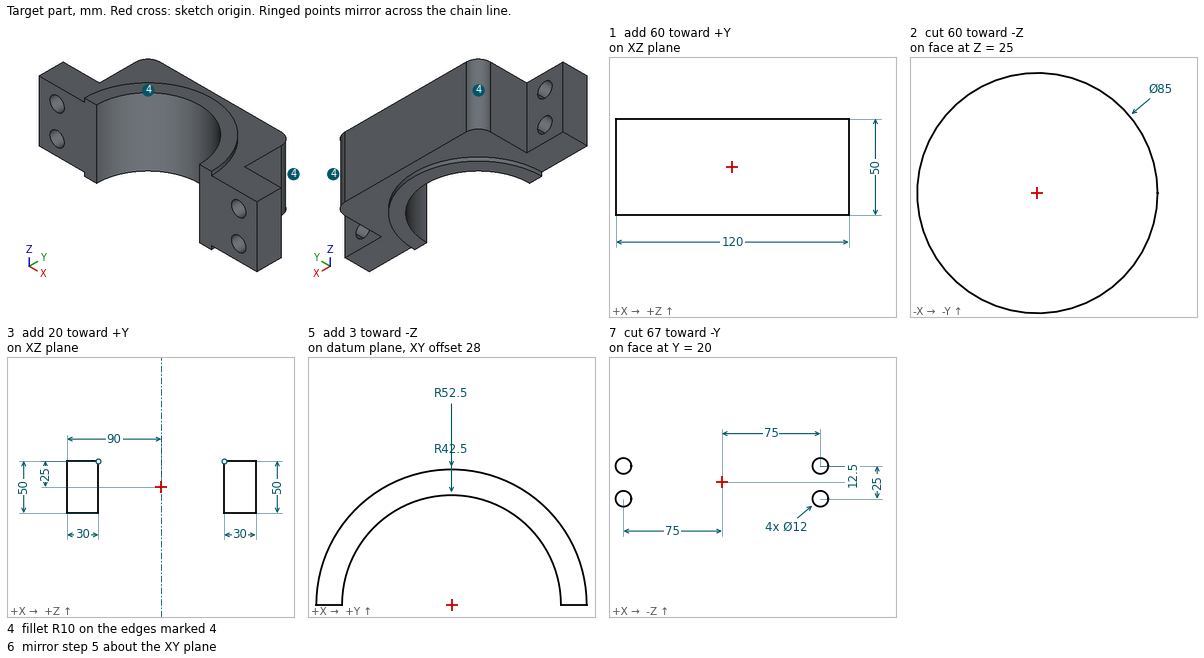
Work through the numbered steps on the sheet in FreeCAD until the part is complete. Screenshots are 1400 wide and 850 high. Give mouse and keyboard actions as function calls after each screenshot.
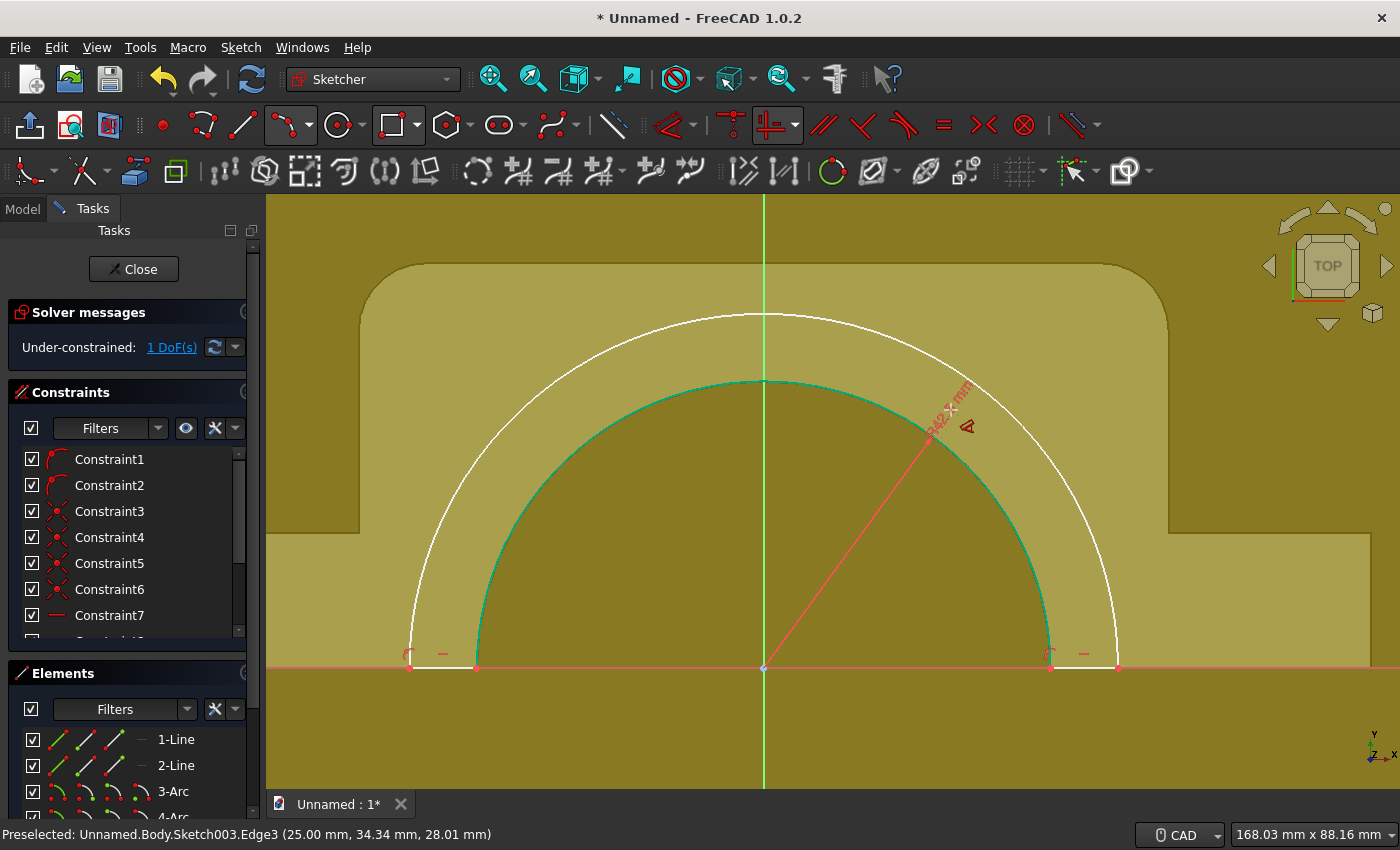
click(972, 382)
click(991, 356)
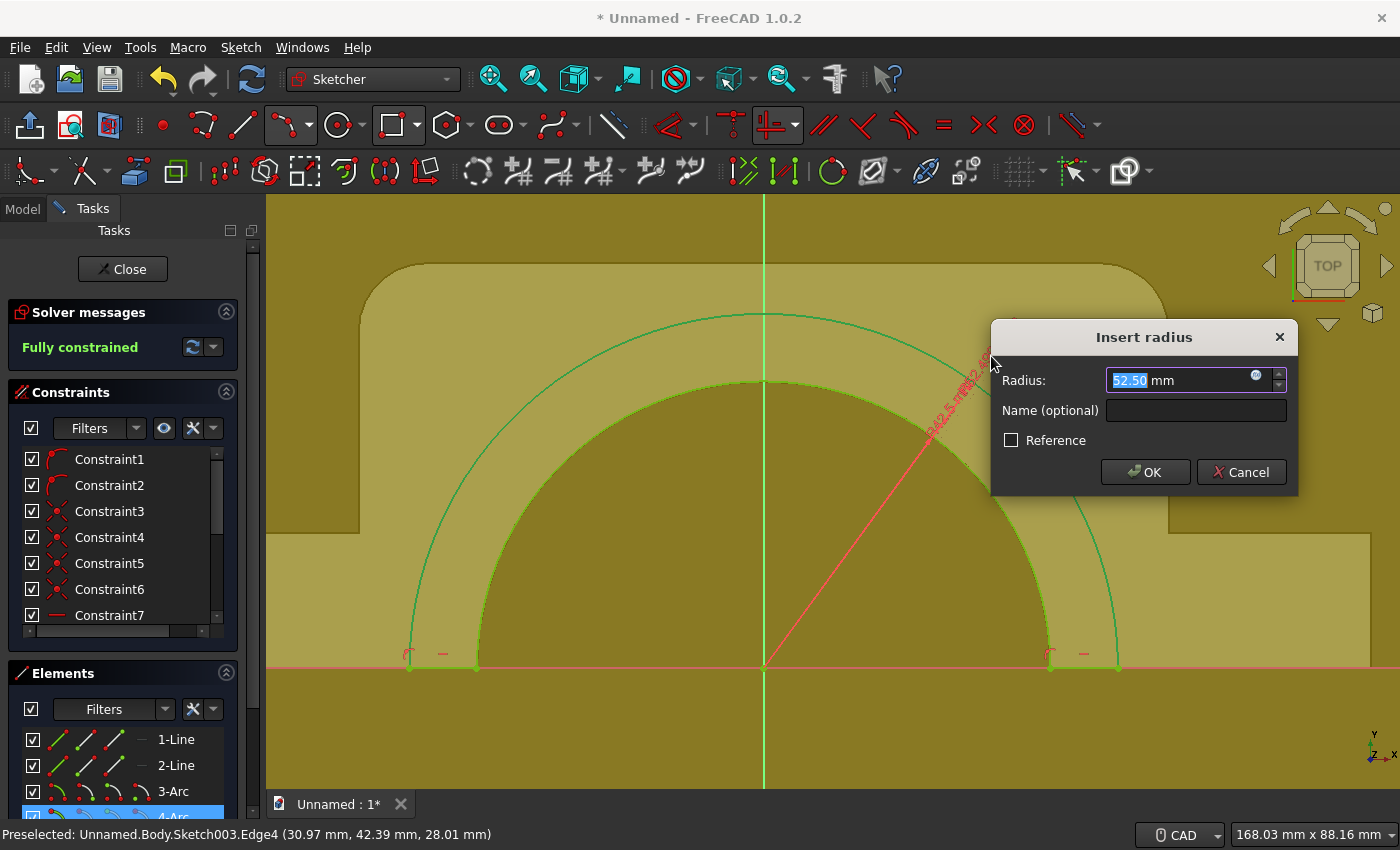
text(52.5)
key(Return)
key(Escape)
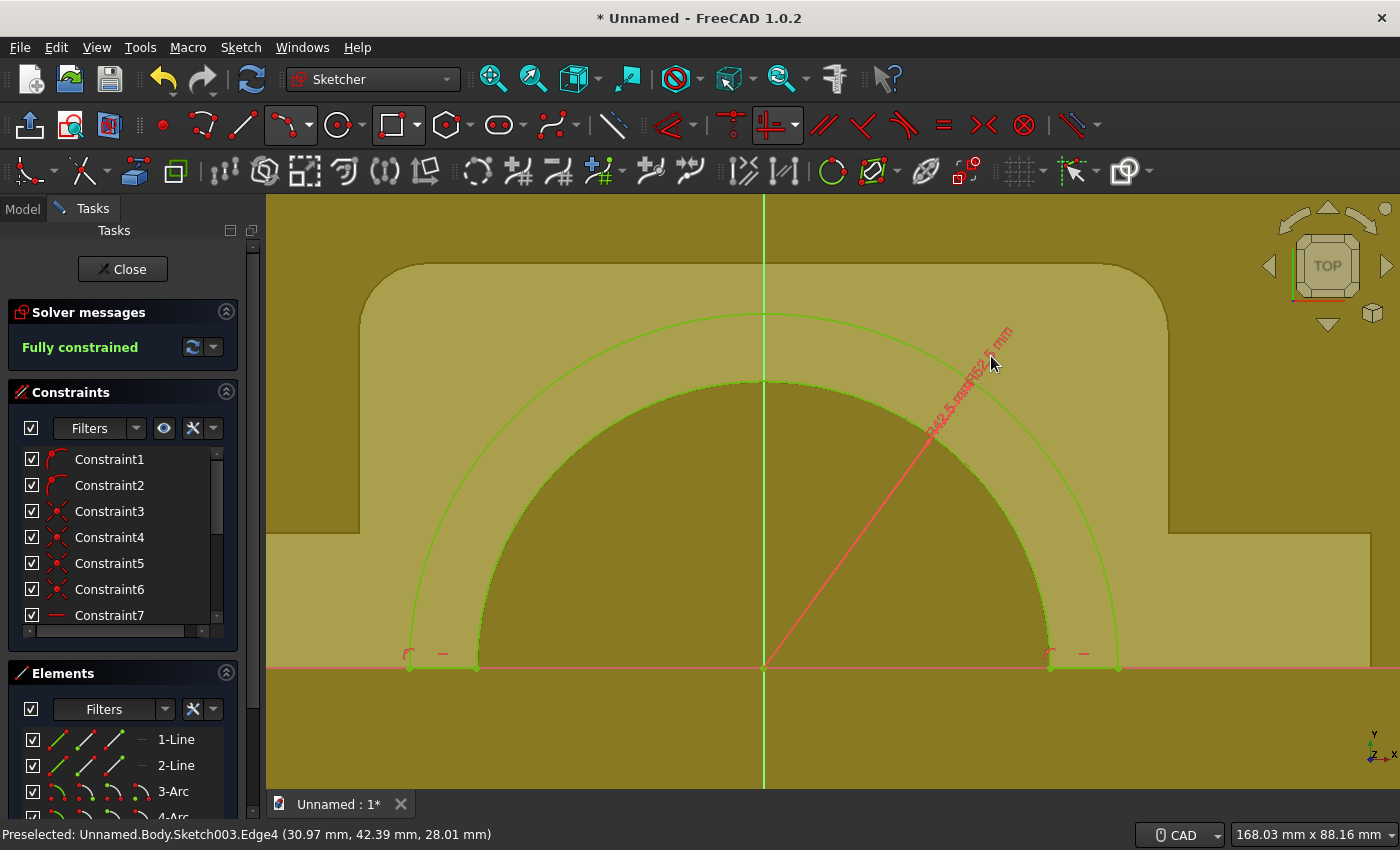
click(123, 269)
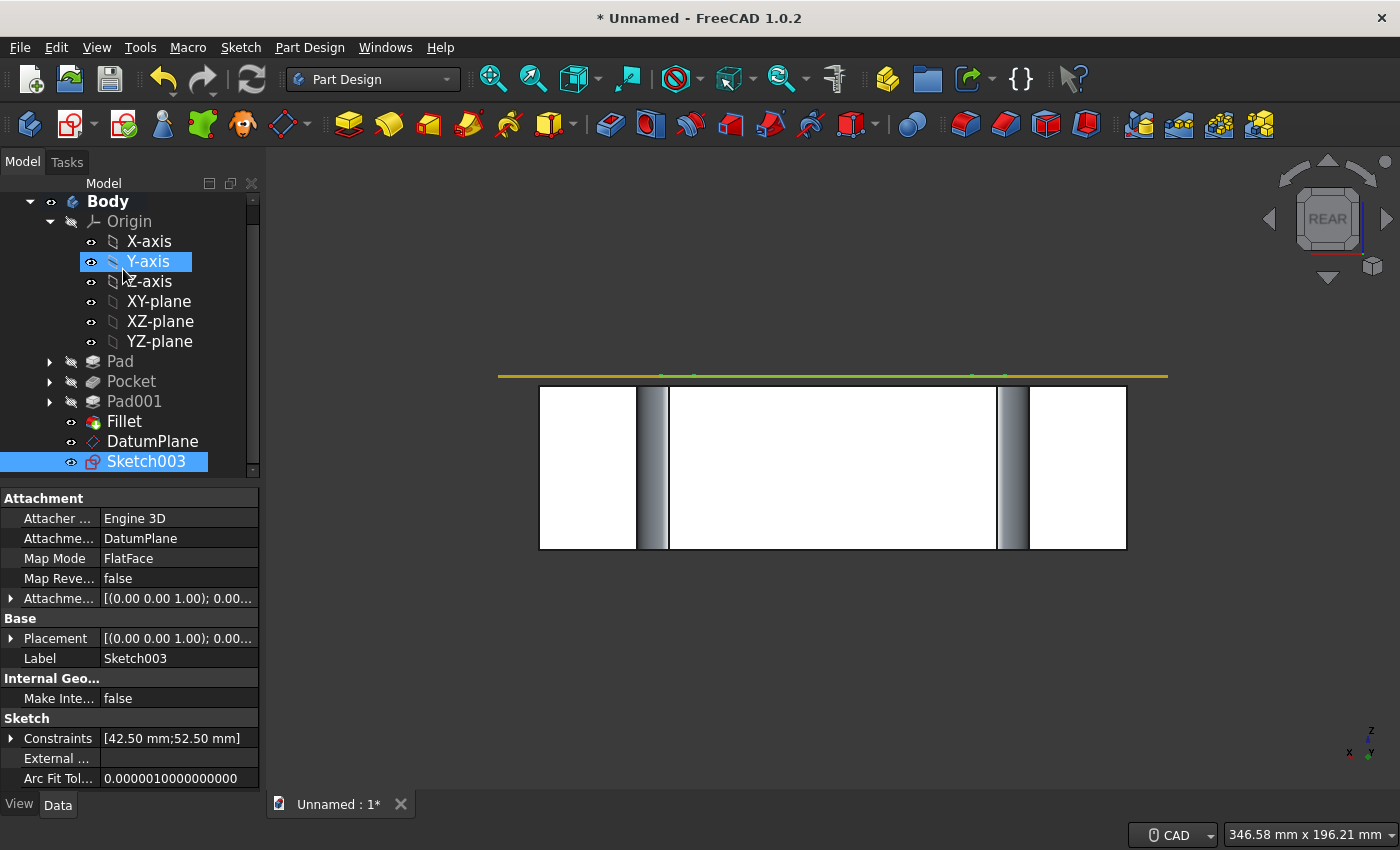
click(350, 124)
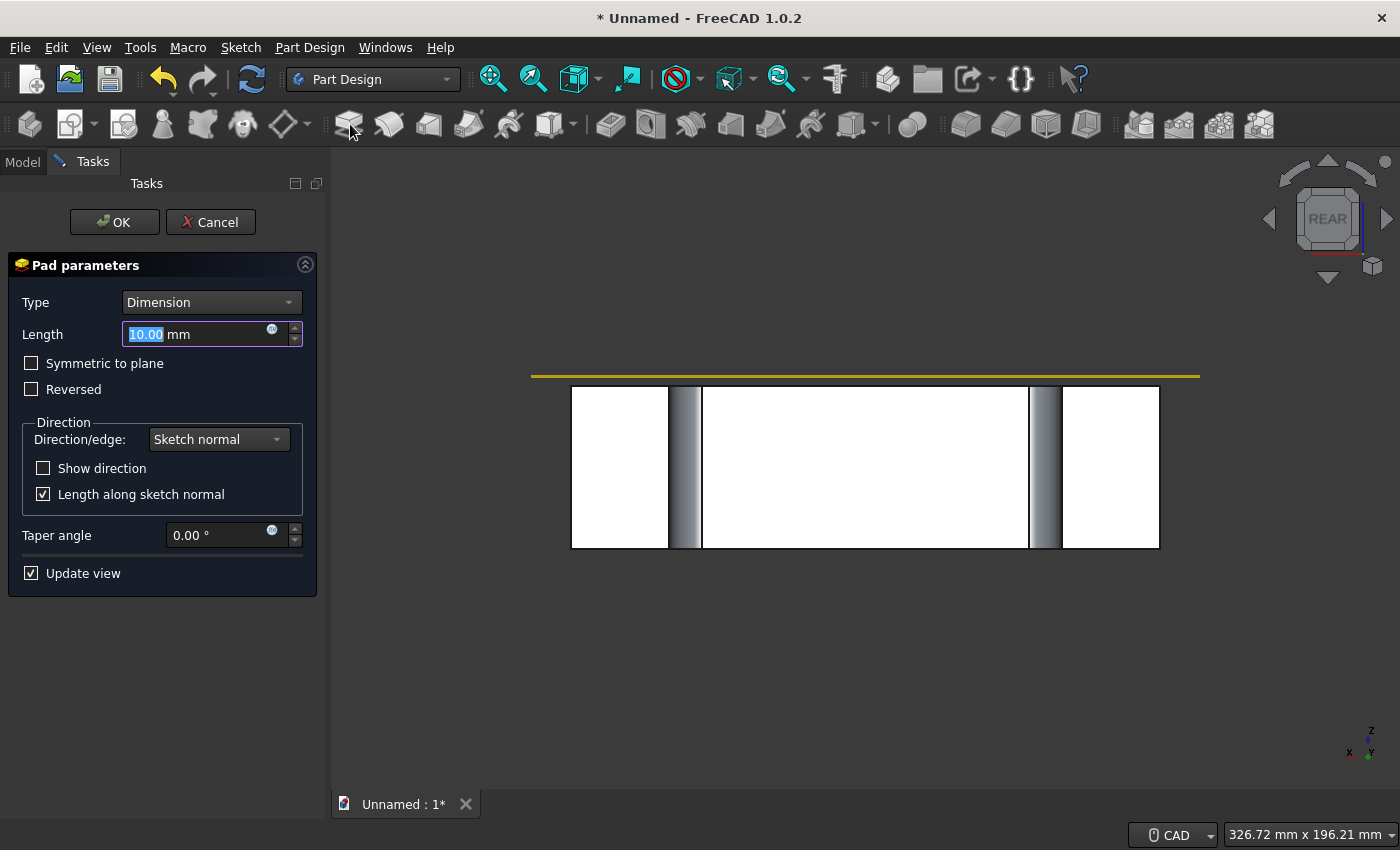
text(3)
key(Tab)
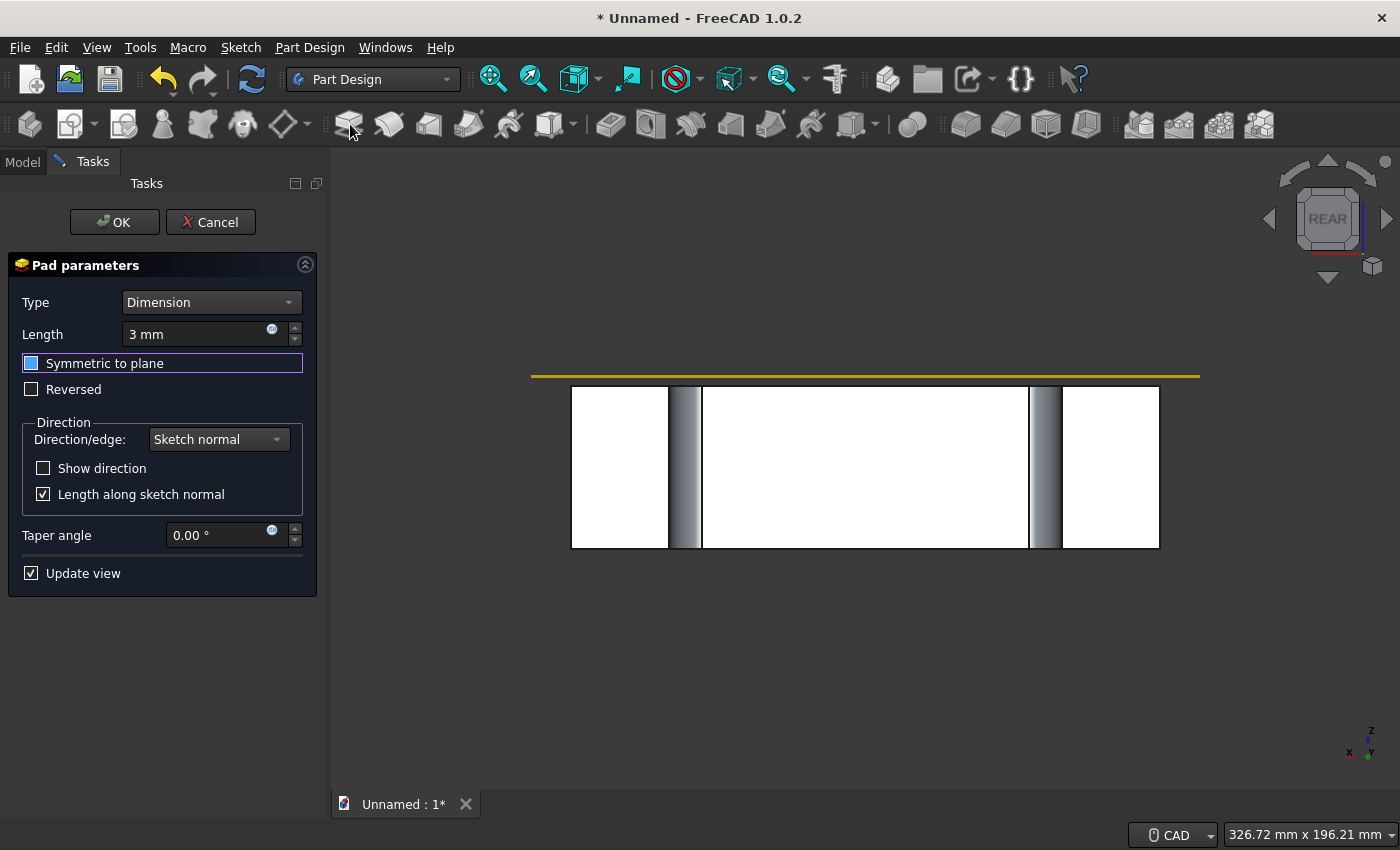
click(30, 389)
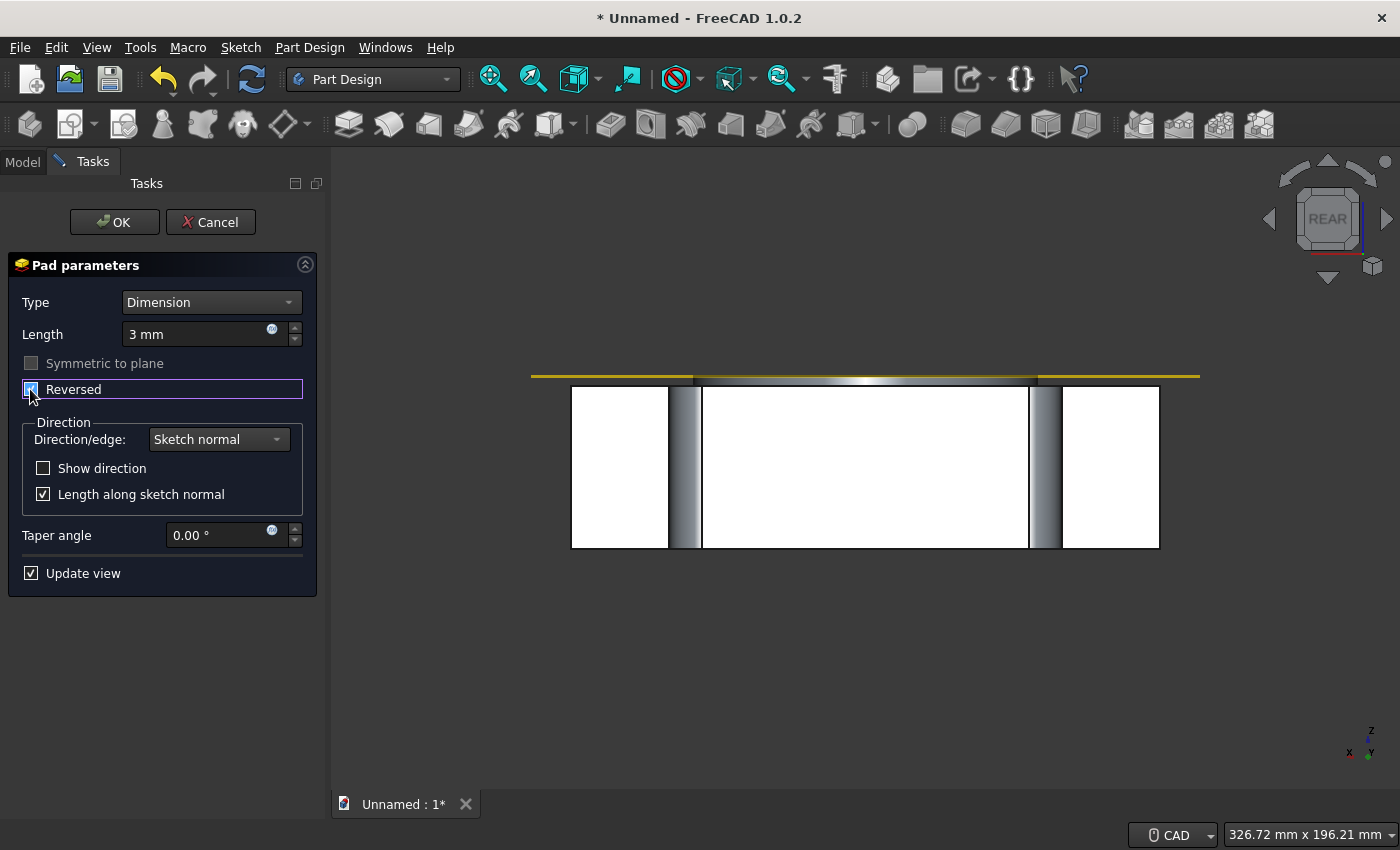
click(115, 222)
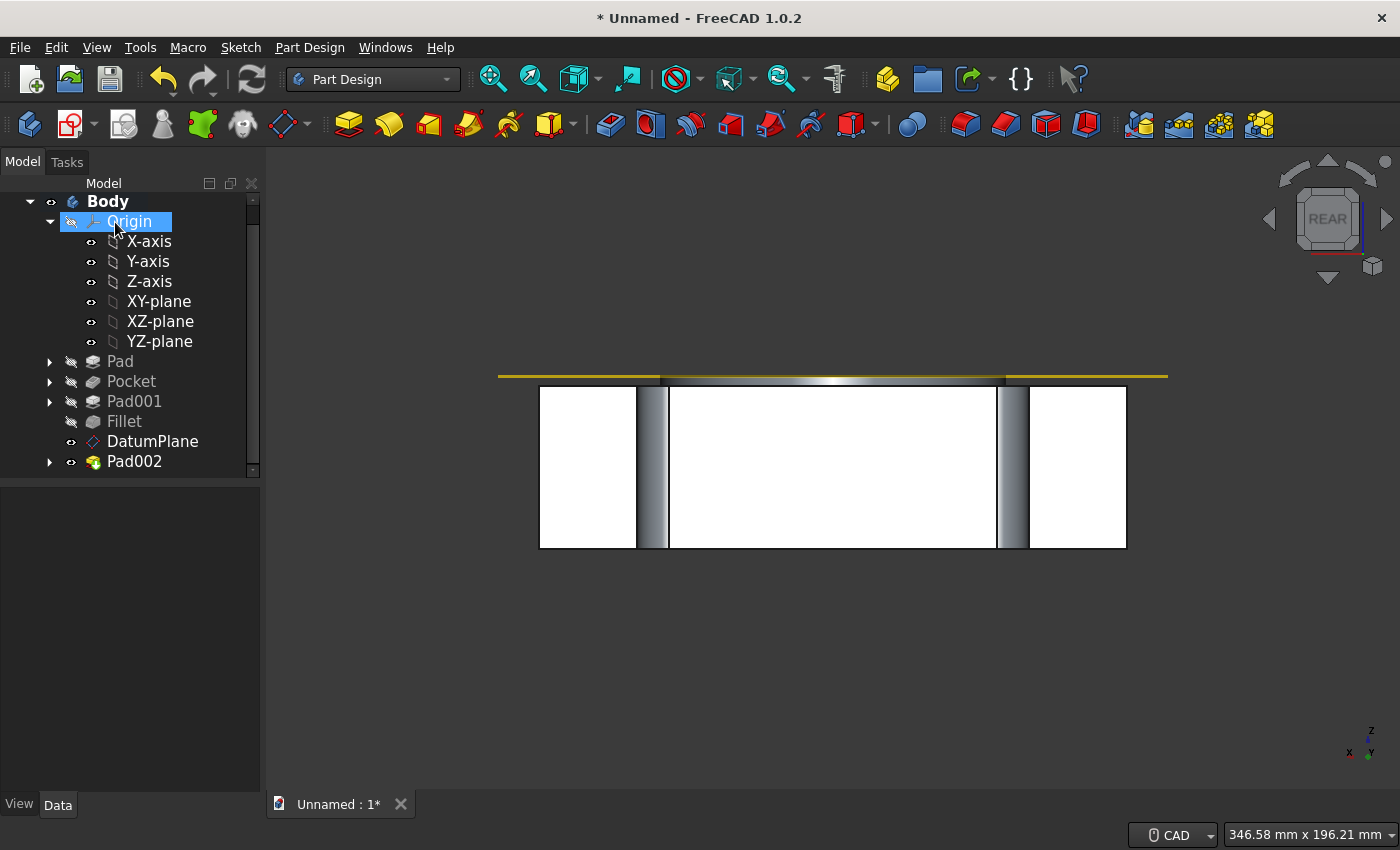
click(116, 442)
key(space)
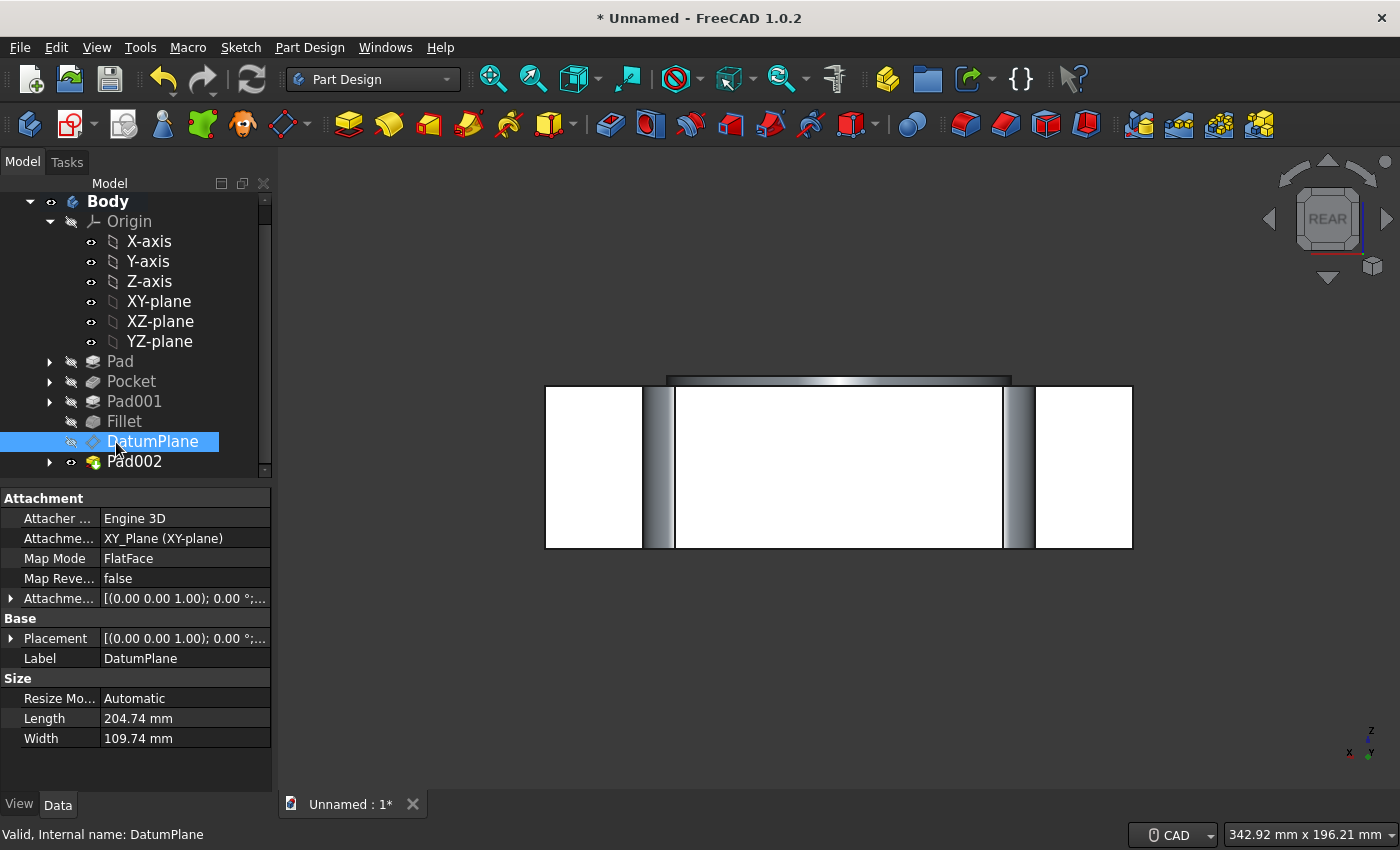
click(116, 462)